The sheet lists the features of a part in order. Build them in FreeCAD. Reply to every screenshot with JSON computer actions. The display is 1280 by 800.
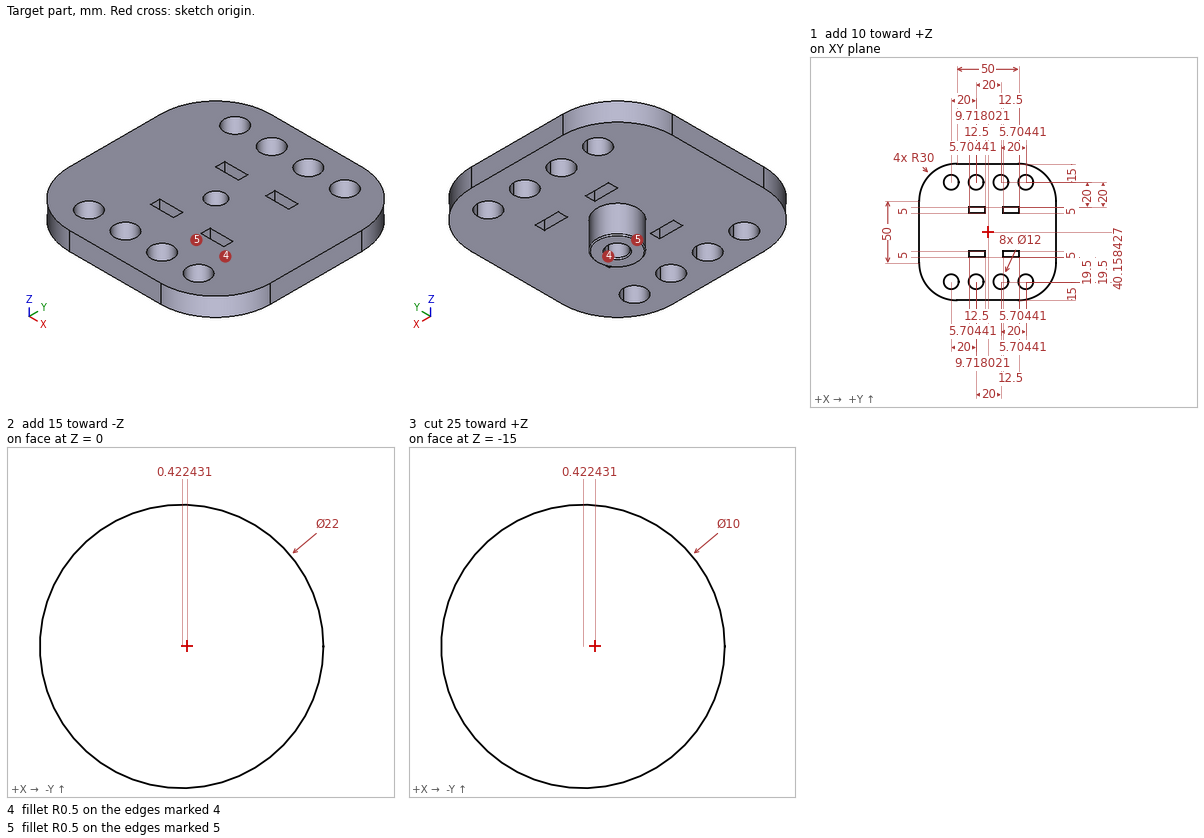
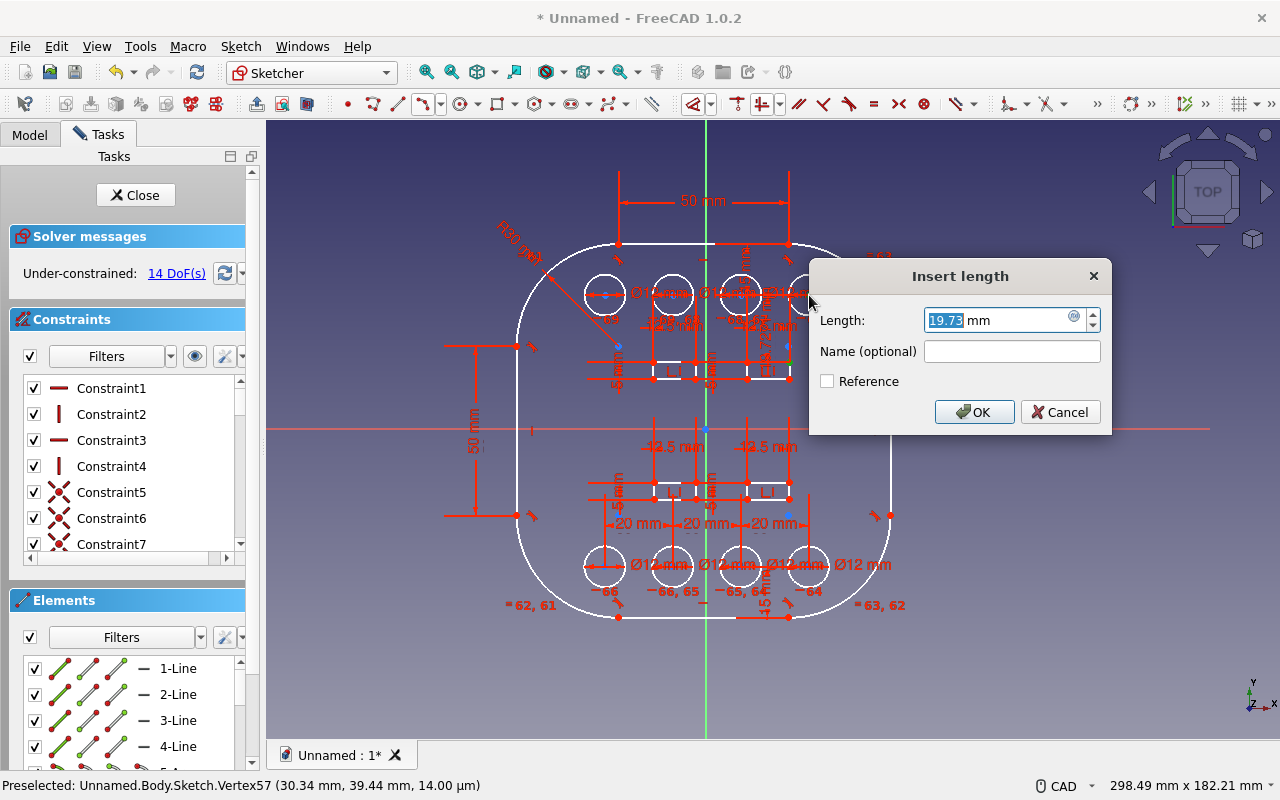
{"action": "type", "text": "20"}
{"action": "key", "text": "Return"}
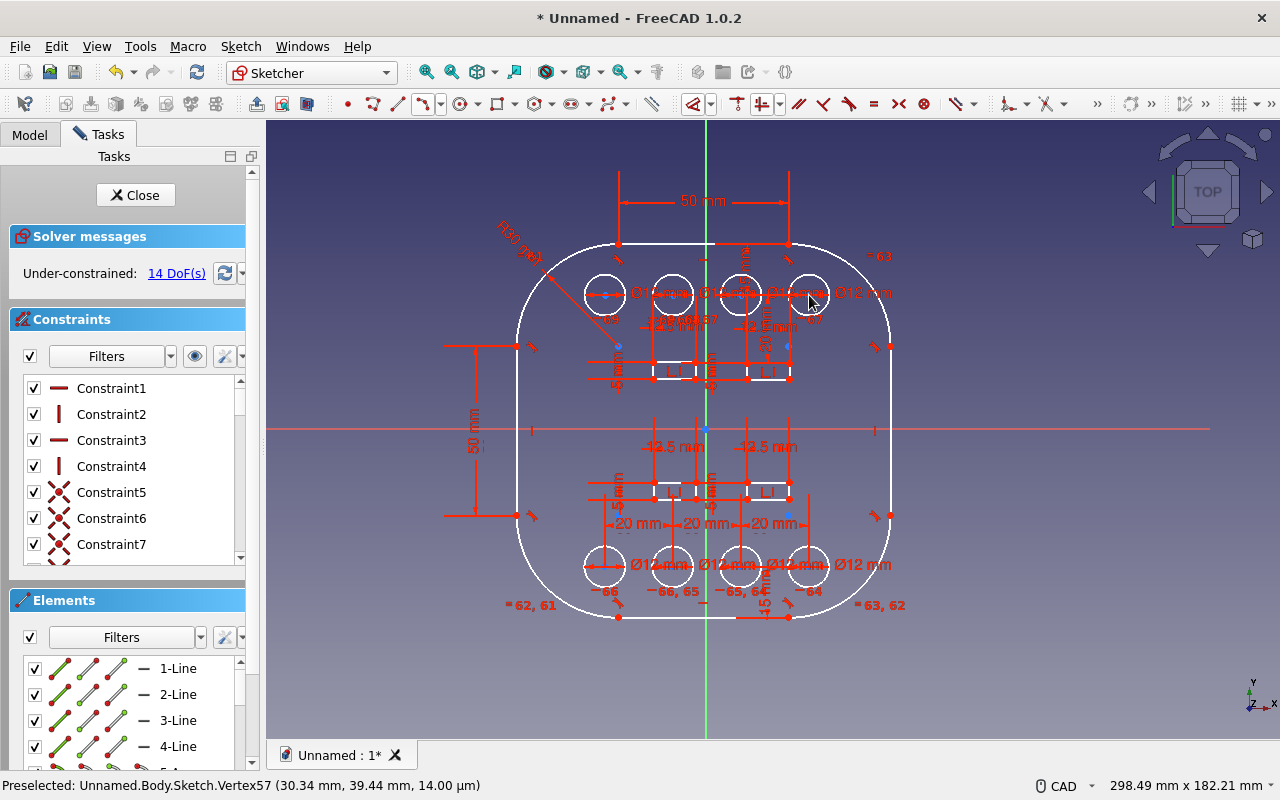
{"action": "left_click", "coordinate": [809, 295]}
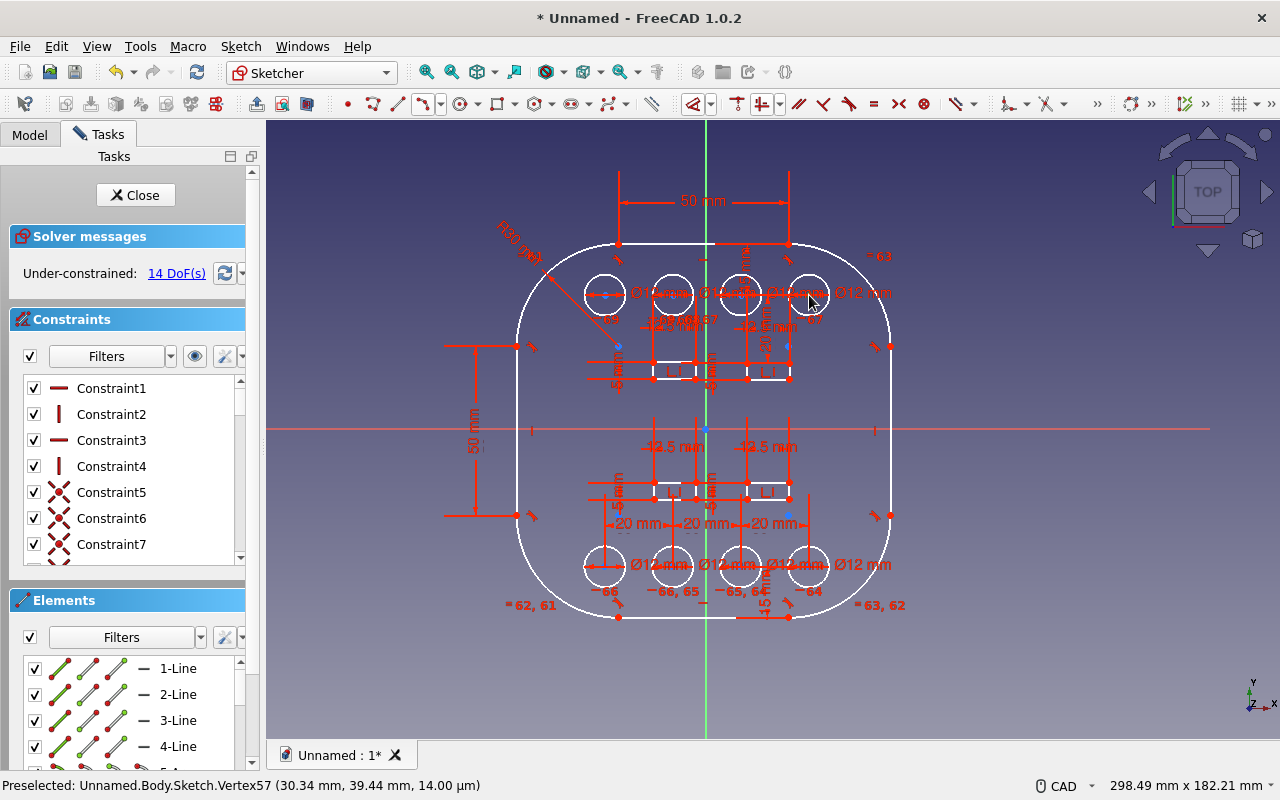
{"action": "left_click", "coordinate": [741, 295]}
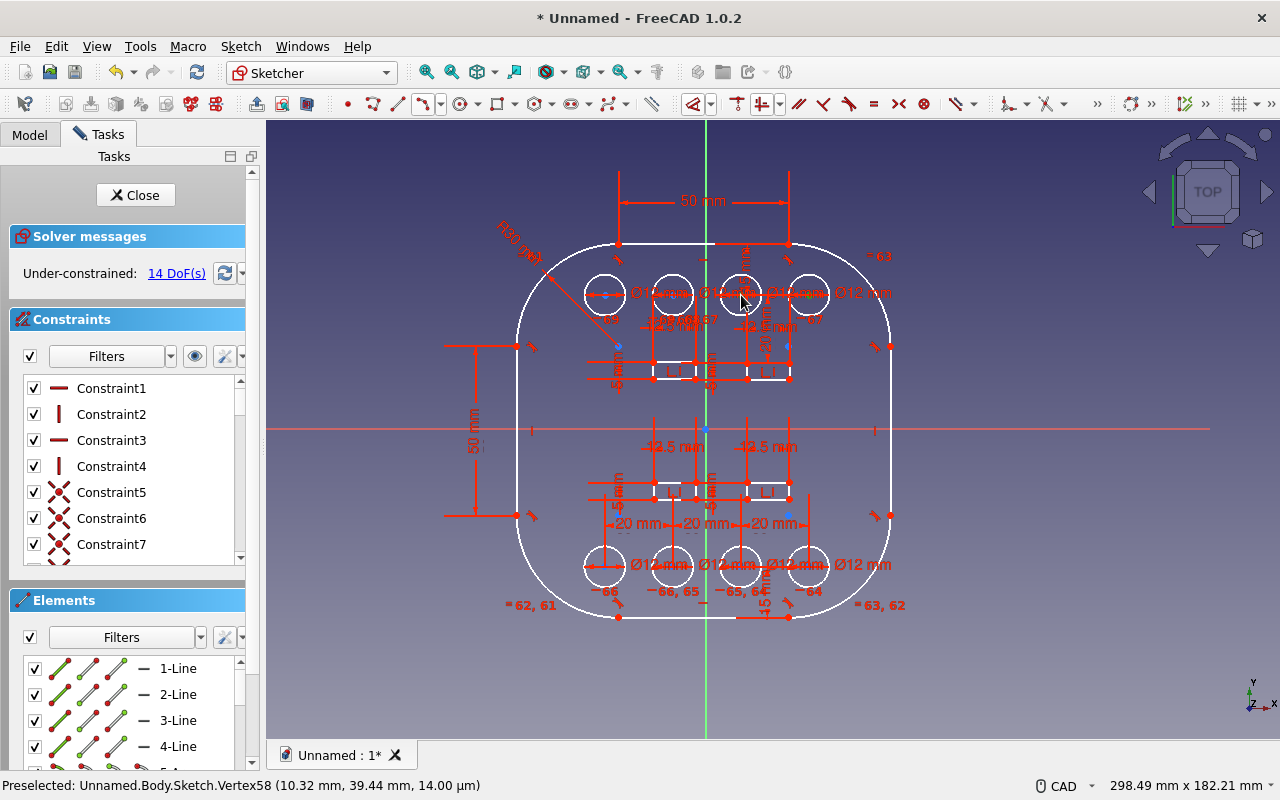
{"action": "key", "text": "l"}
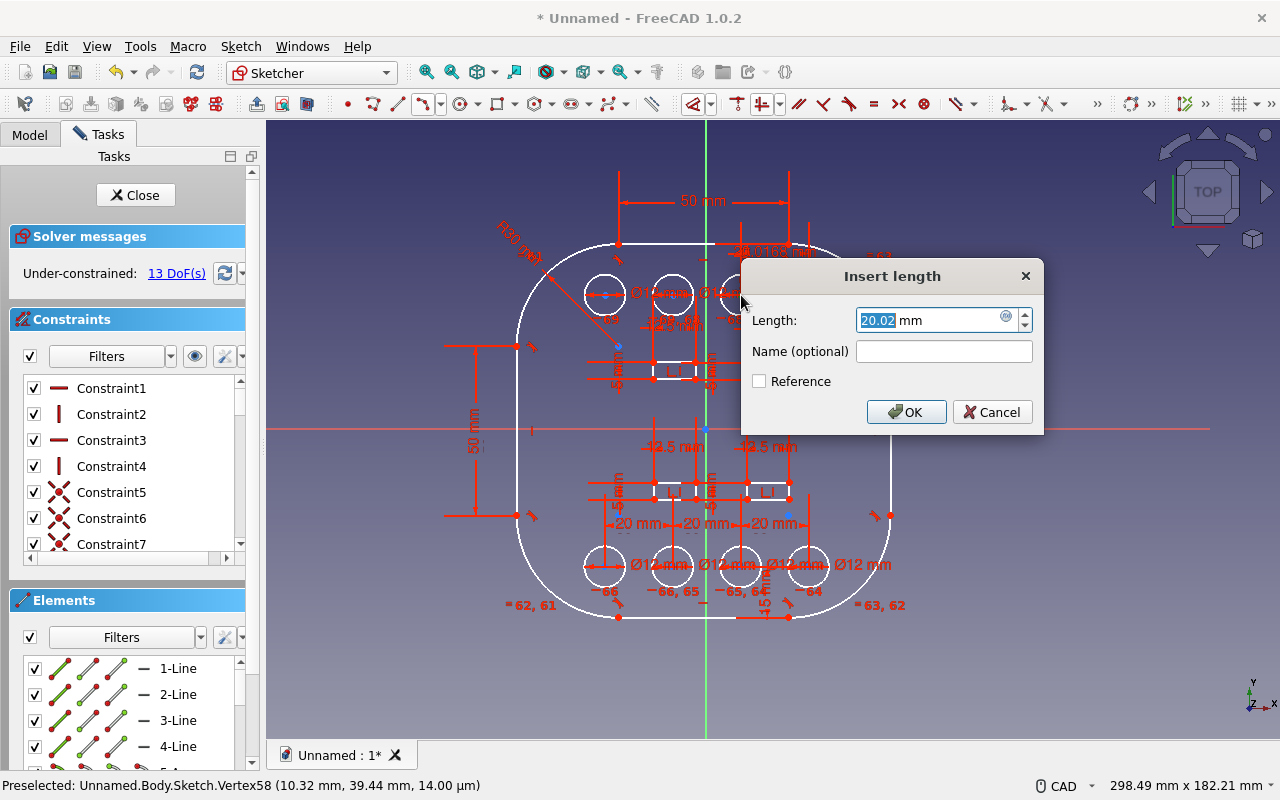
{"action": "type", "text": "20"}
{"action": "key", "text": "Return"}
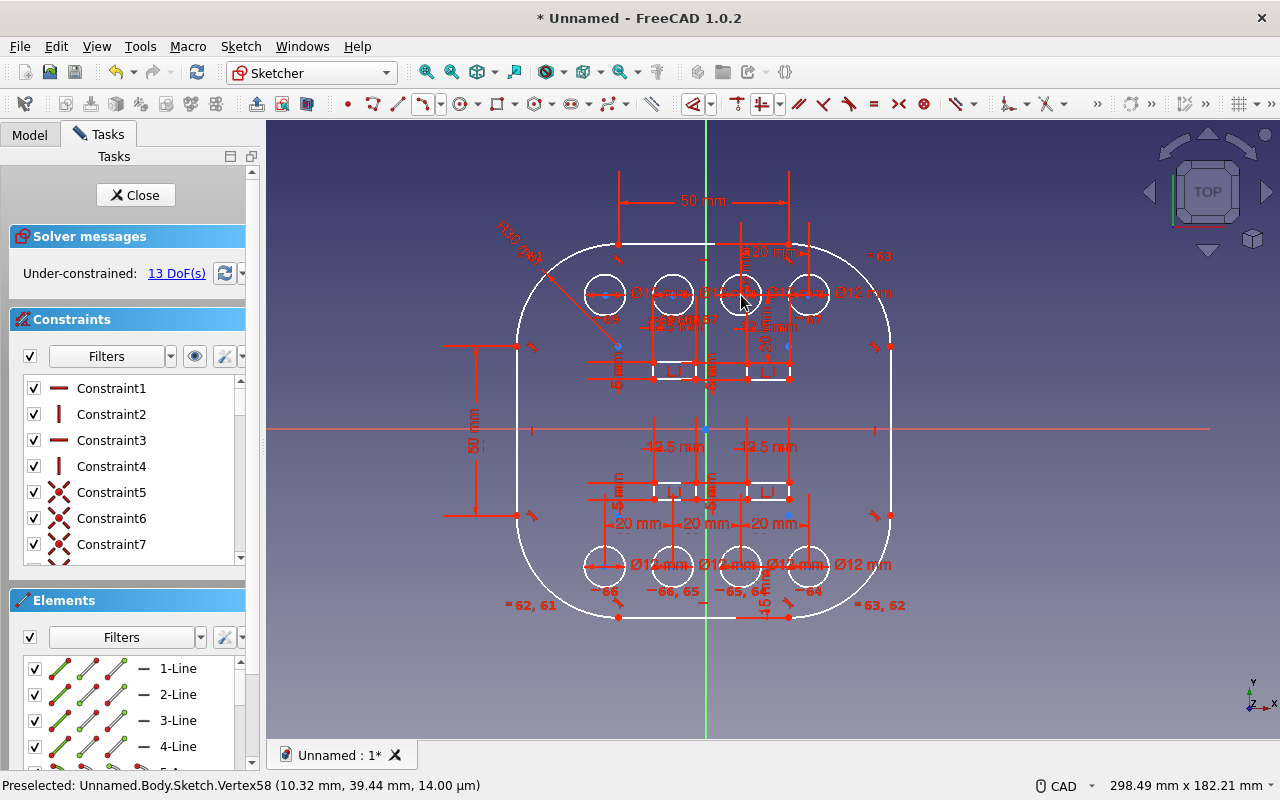
{"action": "left_click", "coordinate": [696, 362]}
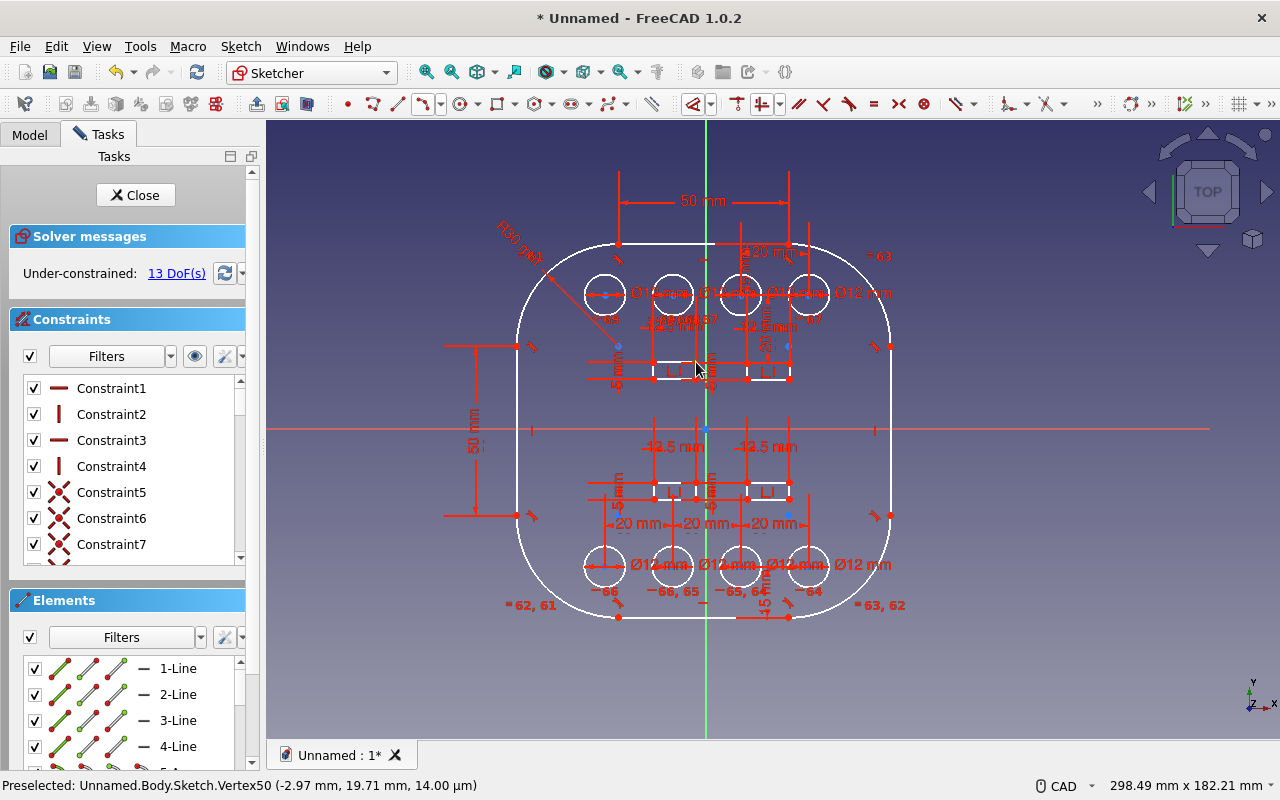
{"action": "left_click", "coordinate": [741, 295]}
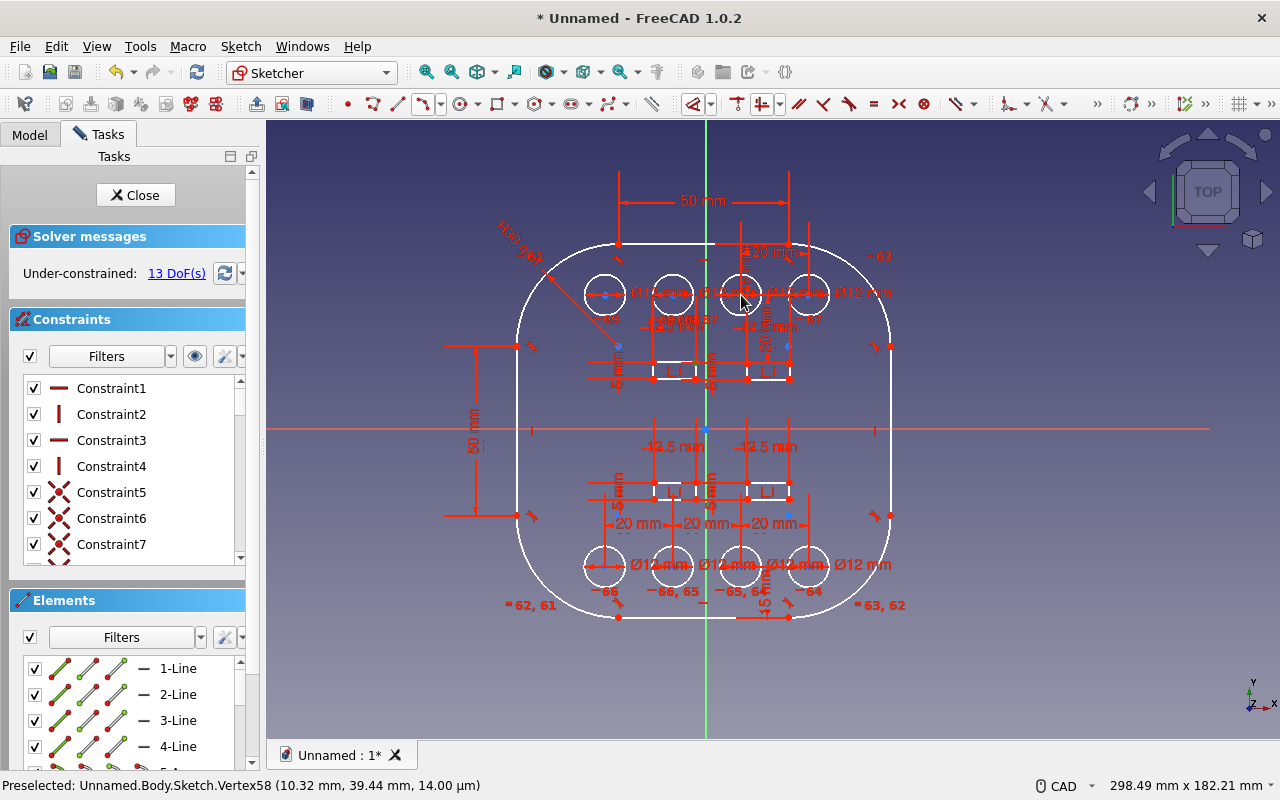
{"action": "left_click", "coordinate": [710, 104]}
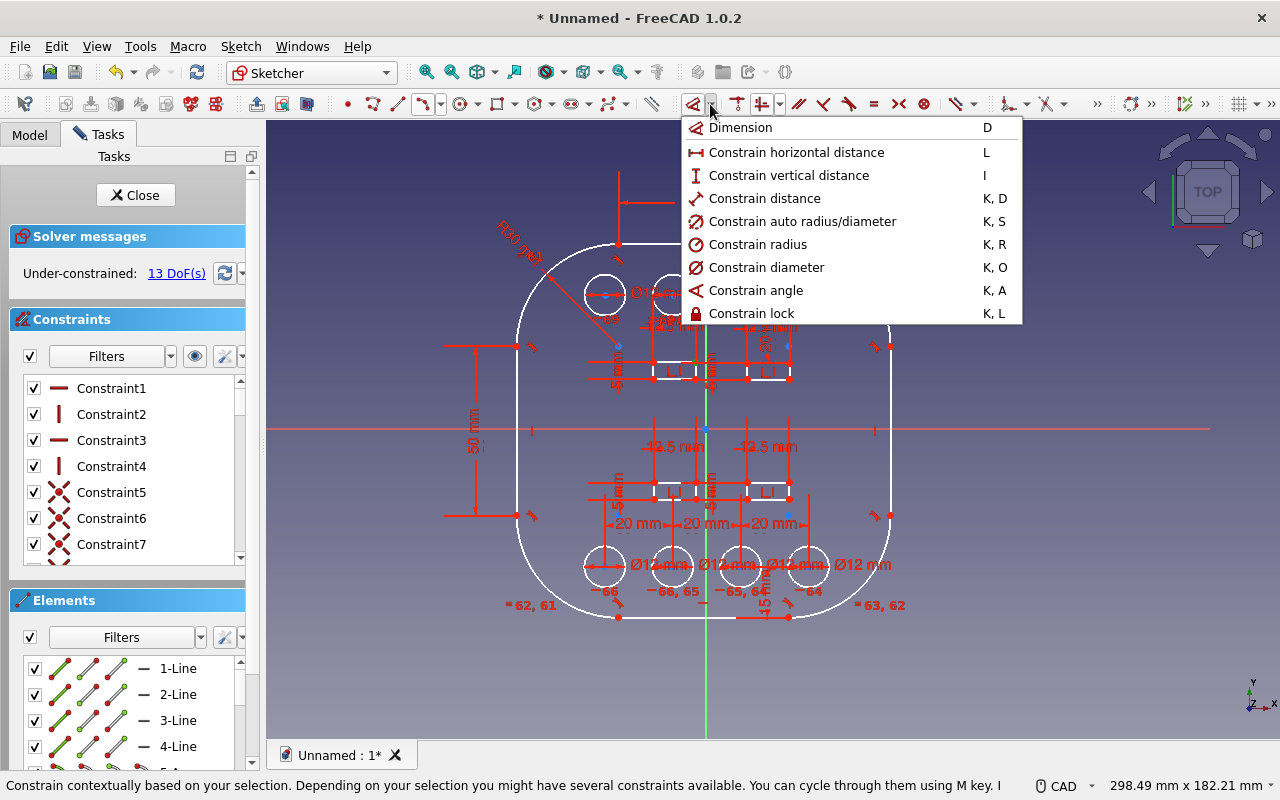
{"action": "left_click", "coordinate": [852, 176]}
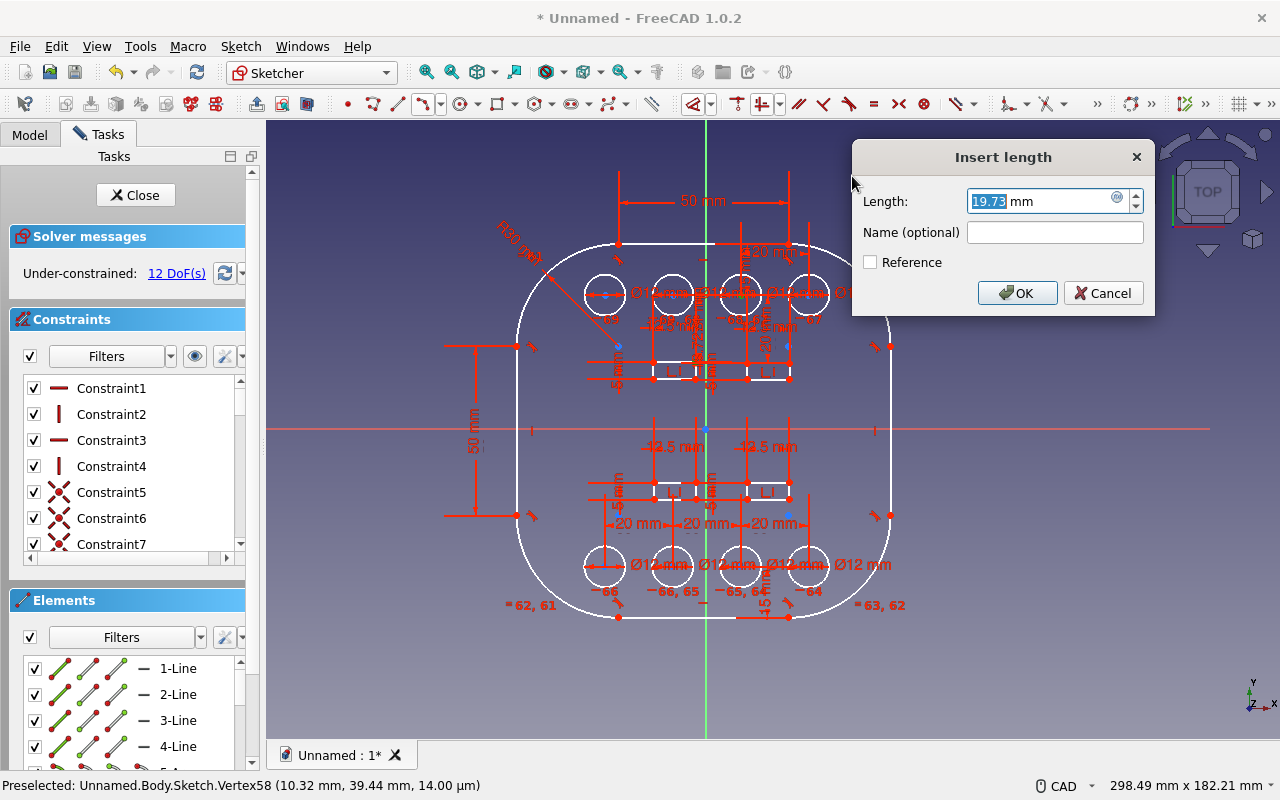
{"action": "type", "text": "20"}
{"action": "key", "text": "Return"}